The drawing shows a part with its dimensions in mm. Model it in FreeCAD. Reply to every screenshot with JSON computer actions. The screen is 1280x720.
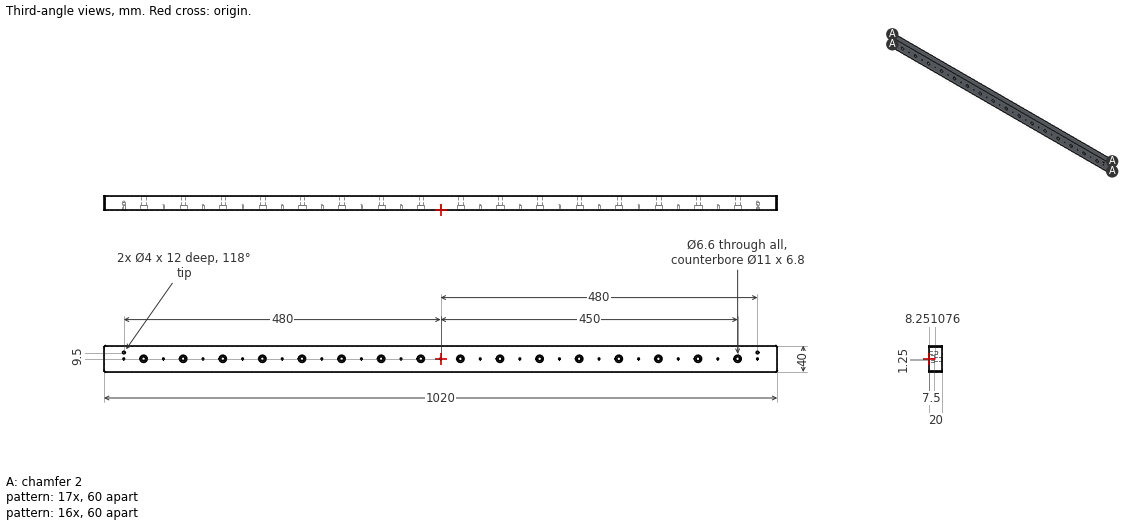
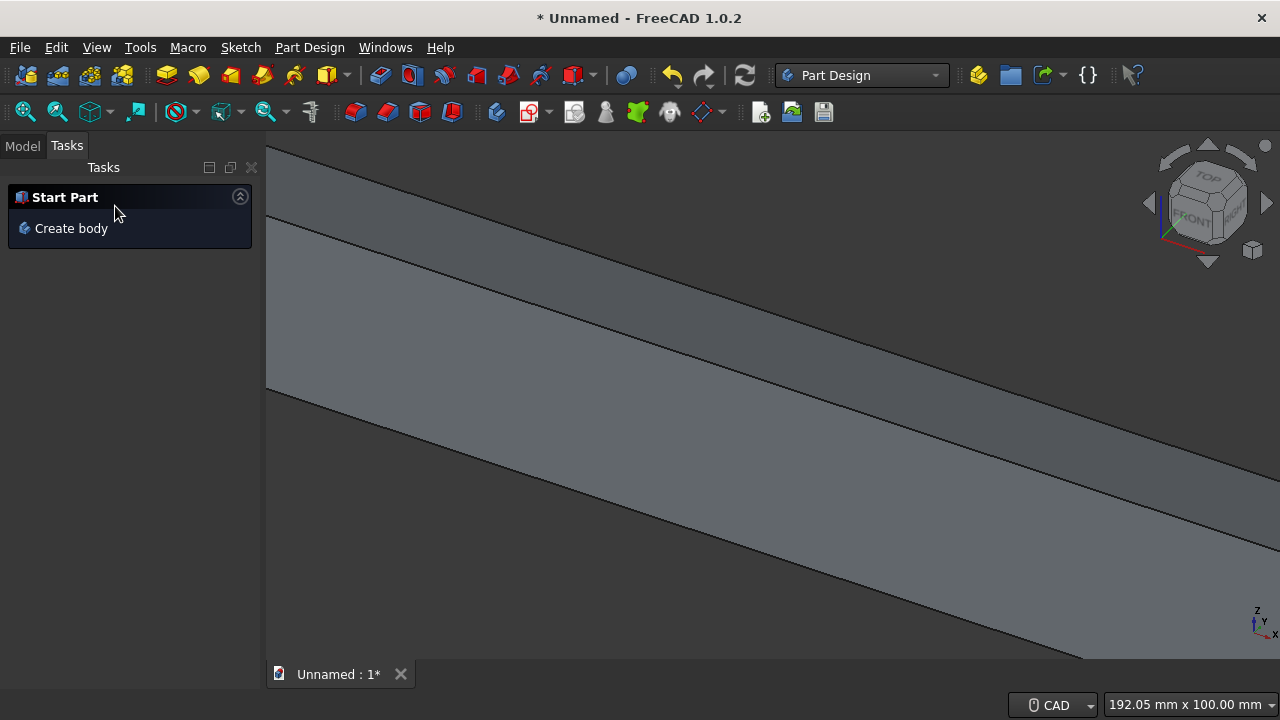
{"action": "left_click", "coordinate": [26, 112]}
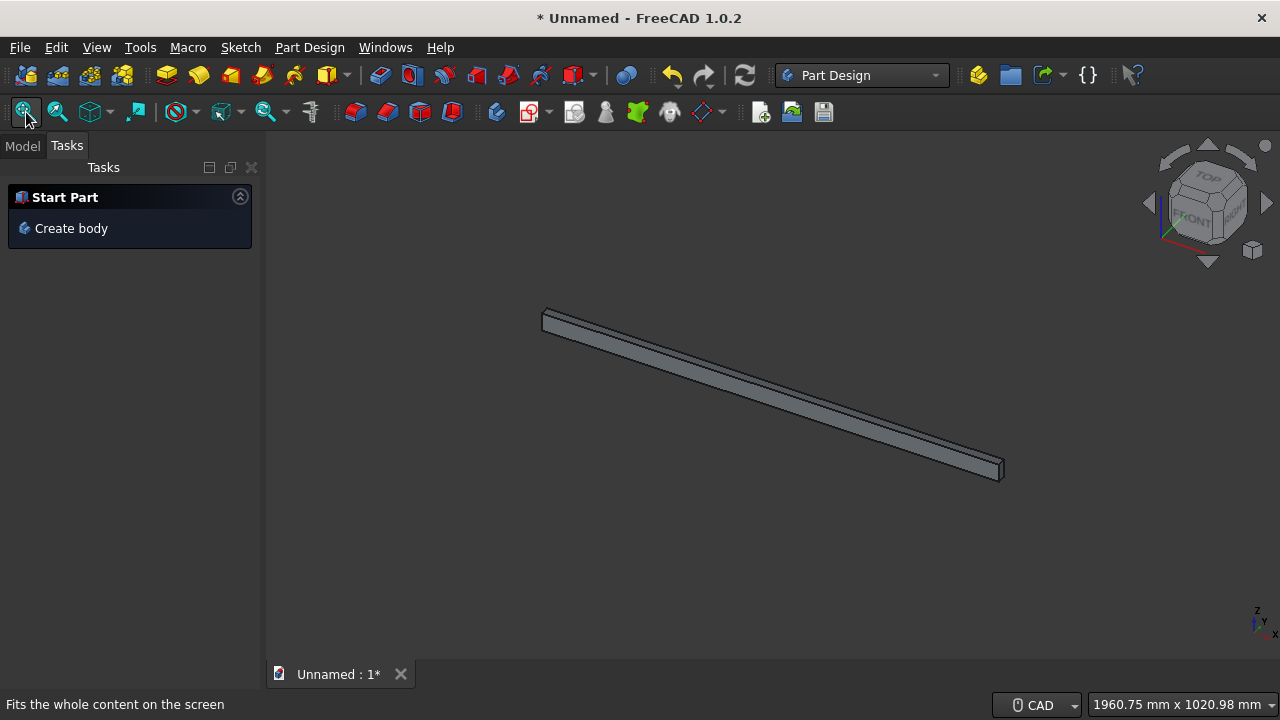
{"action": "scroll", "coordinate": [1001, 461], "scroll_direction": "up", "scroll_amount": 7}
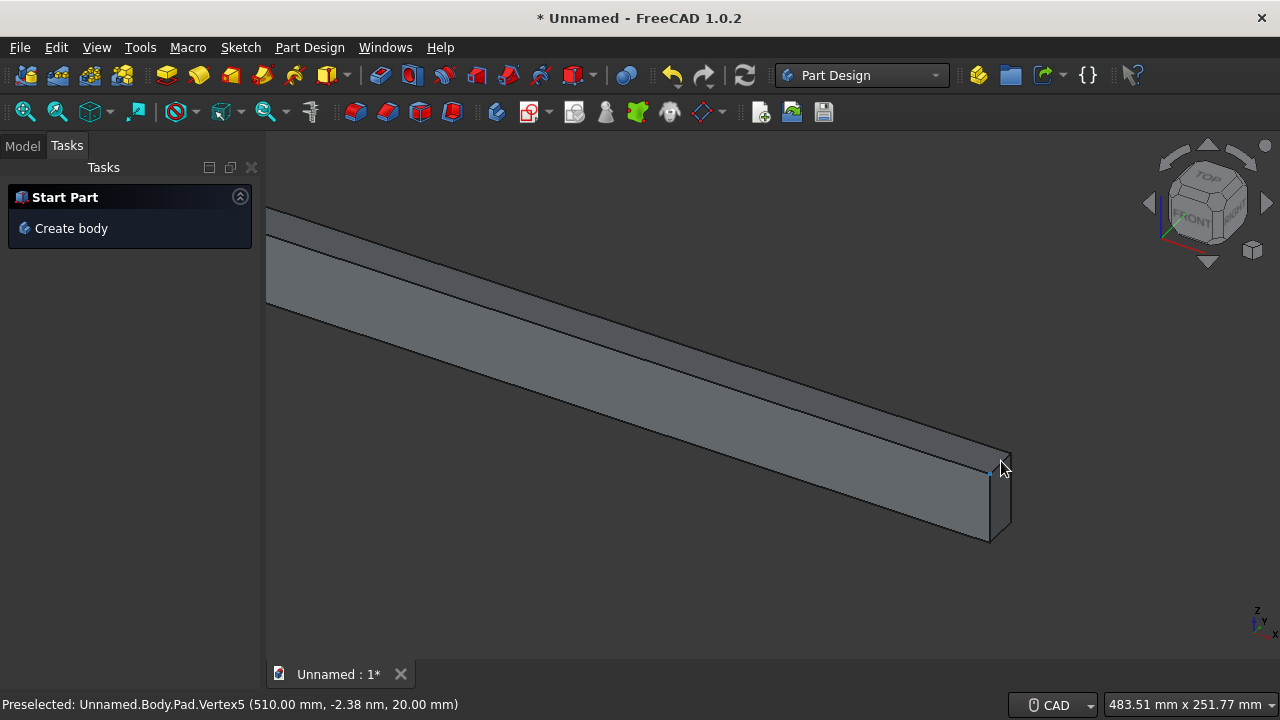
{"action": "left_click", "coordinate": [1000, 463]}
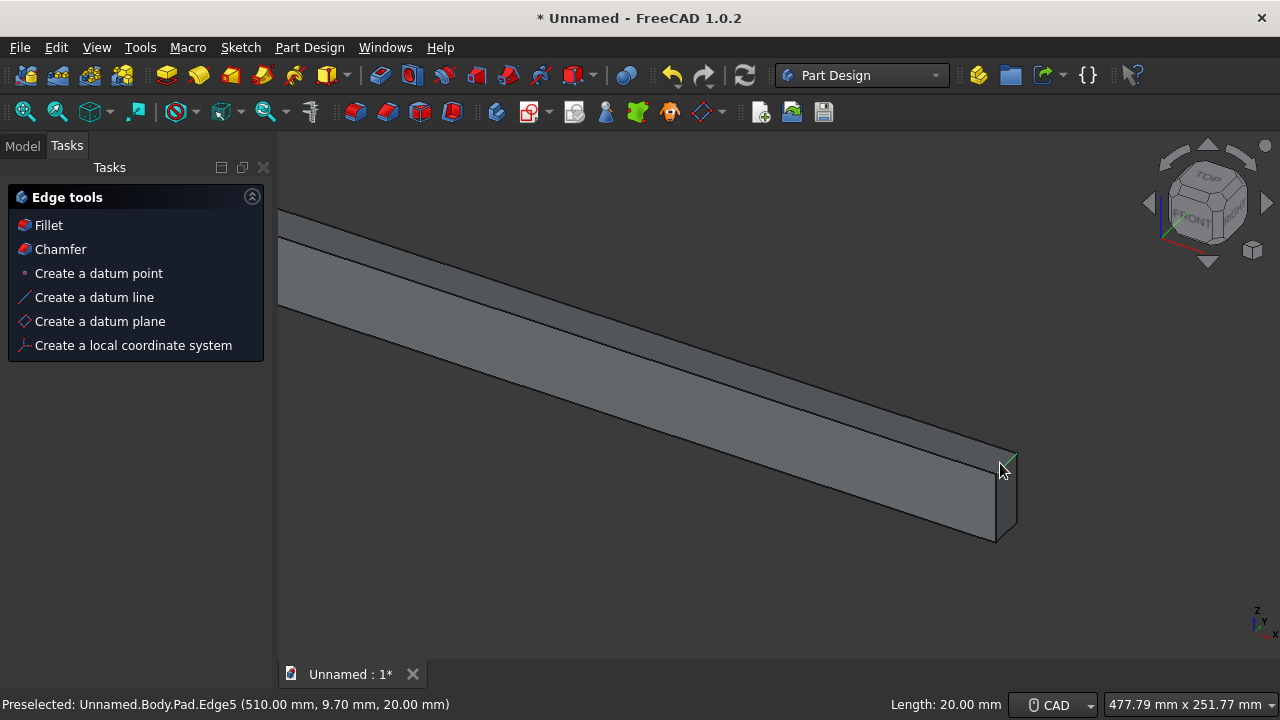
{"action": "key", "text": "v f"}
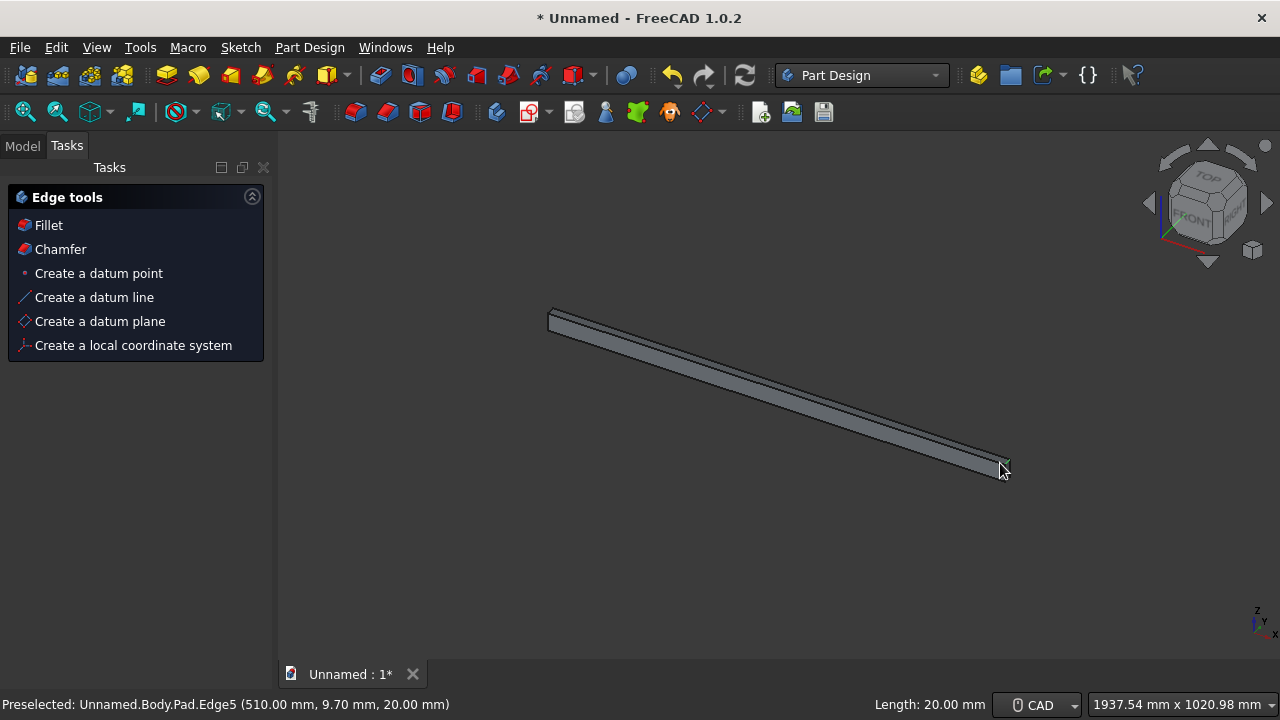
{"action": "key", "text": "0"}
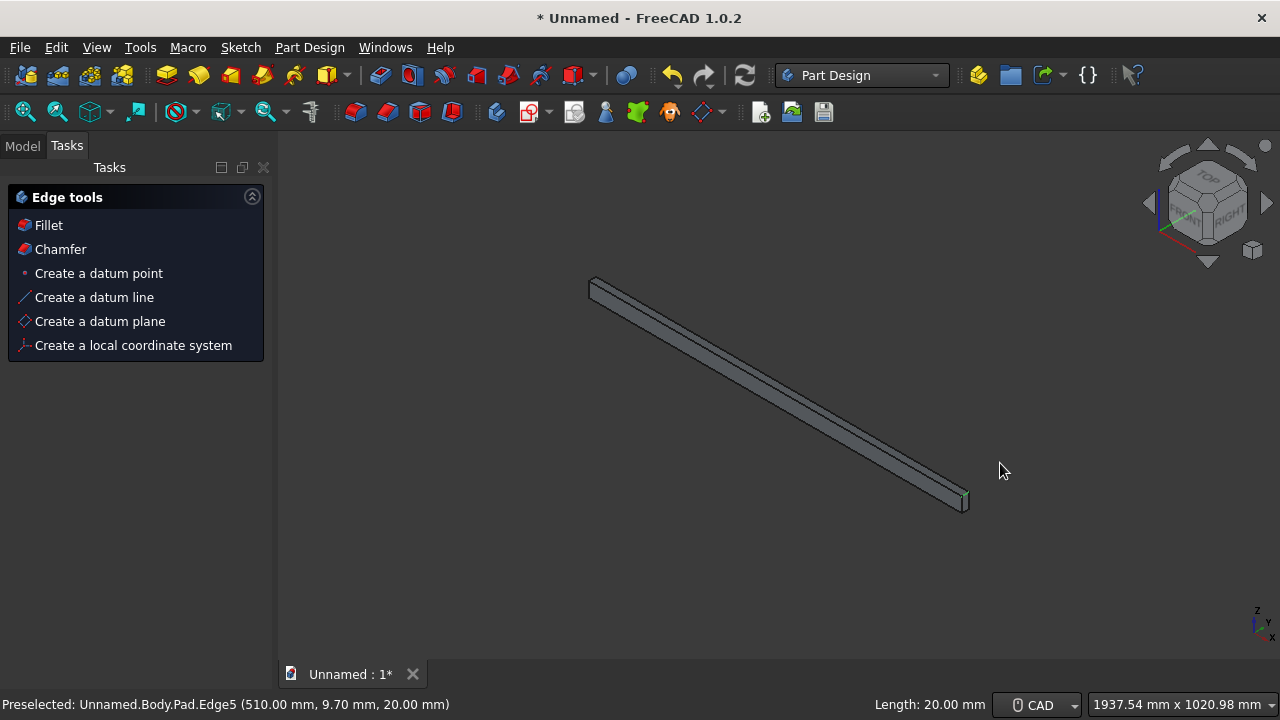
{"action": "key", "text": "v f"}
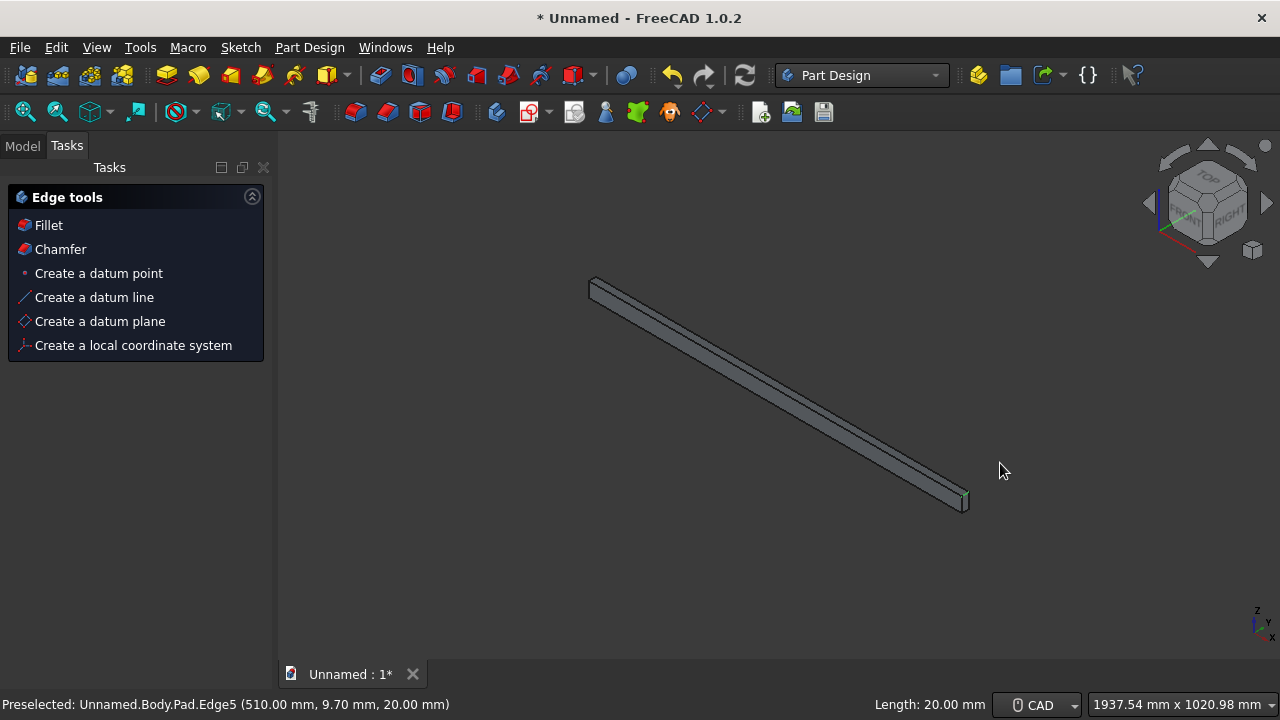
{"action": "scroll", "coordinate": [593, 278], "scroll_direction": "up", "scroll_amount": 7}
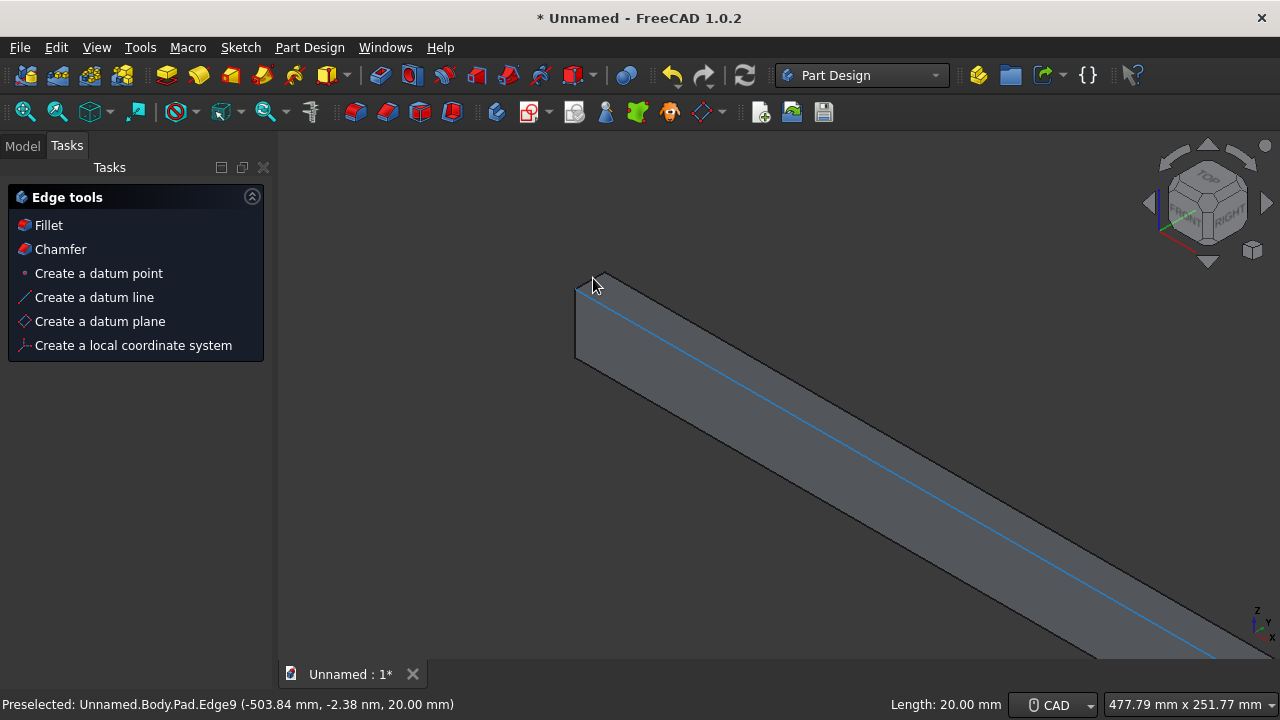
{"action": "key", "text": "v f"}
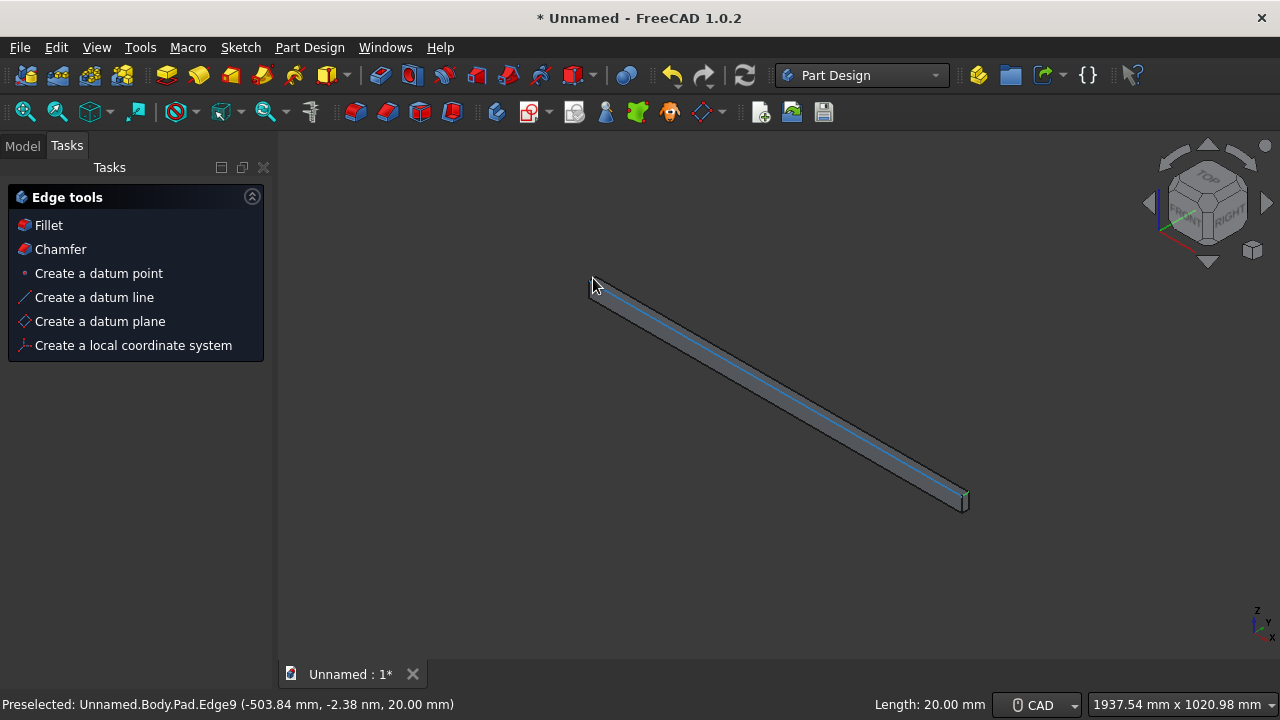
{"action": "key", "text": "2"}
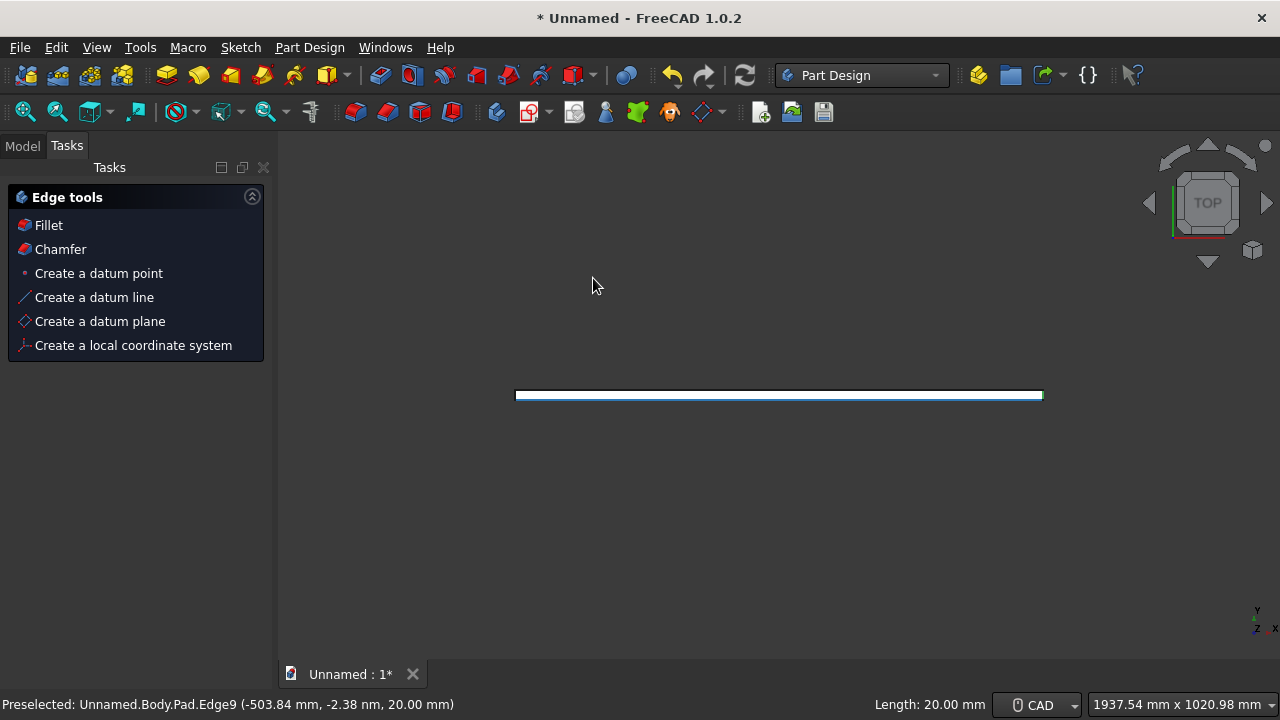
{"action": "left_click", "coordinate": [515, 395], "text": "ctrl"}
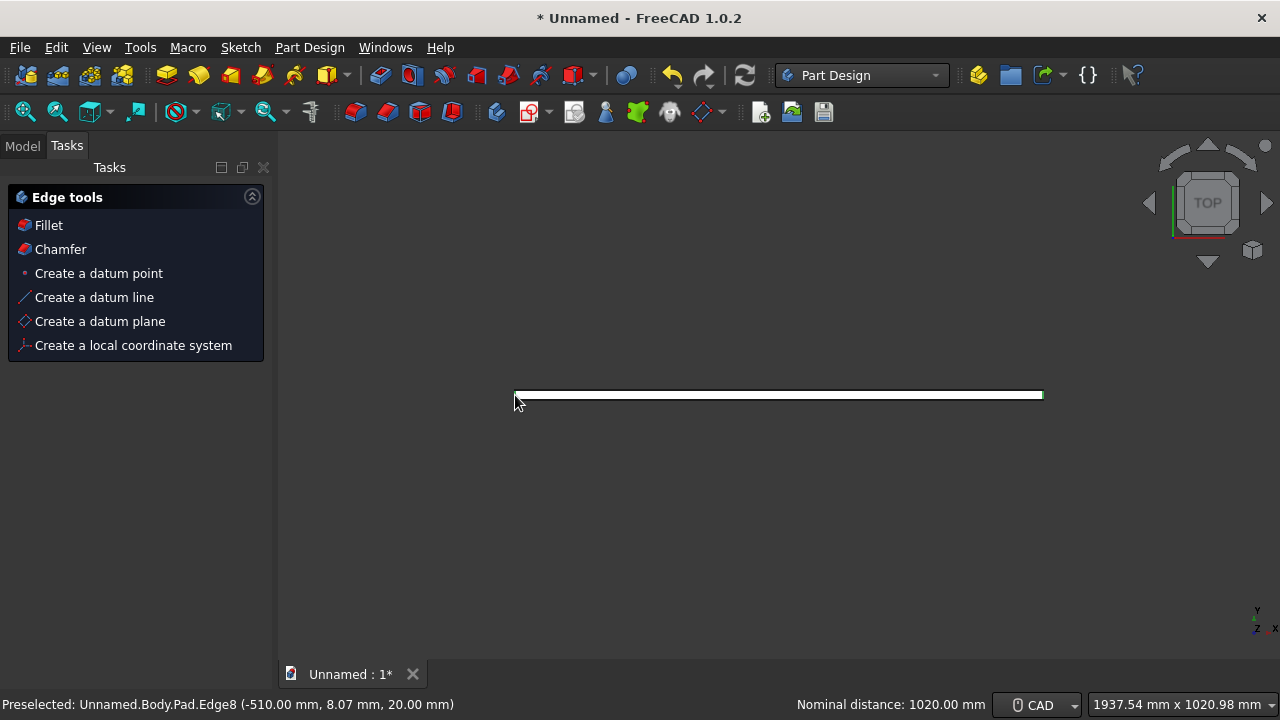
{"action": "scroll", "coordinate": [515, 394], "scroll_direction": "up", "scroll_amount": 7}